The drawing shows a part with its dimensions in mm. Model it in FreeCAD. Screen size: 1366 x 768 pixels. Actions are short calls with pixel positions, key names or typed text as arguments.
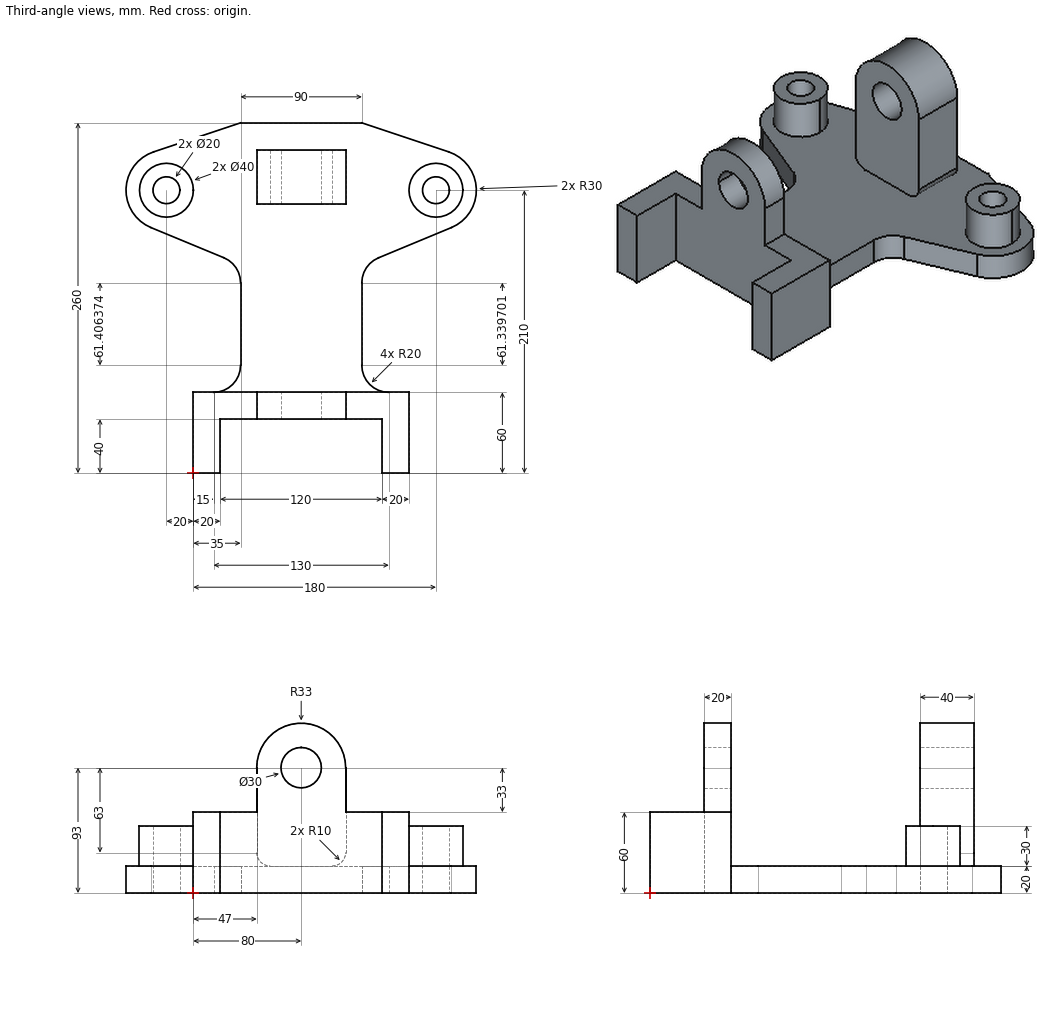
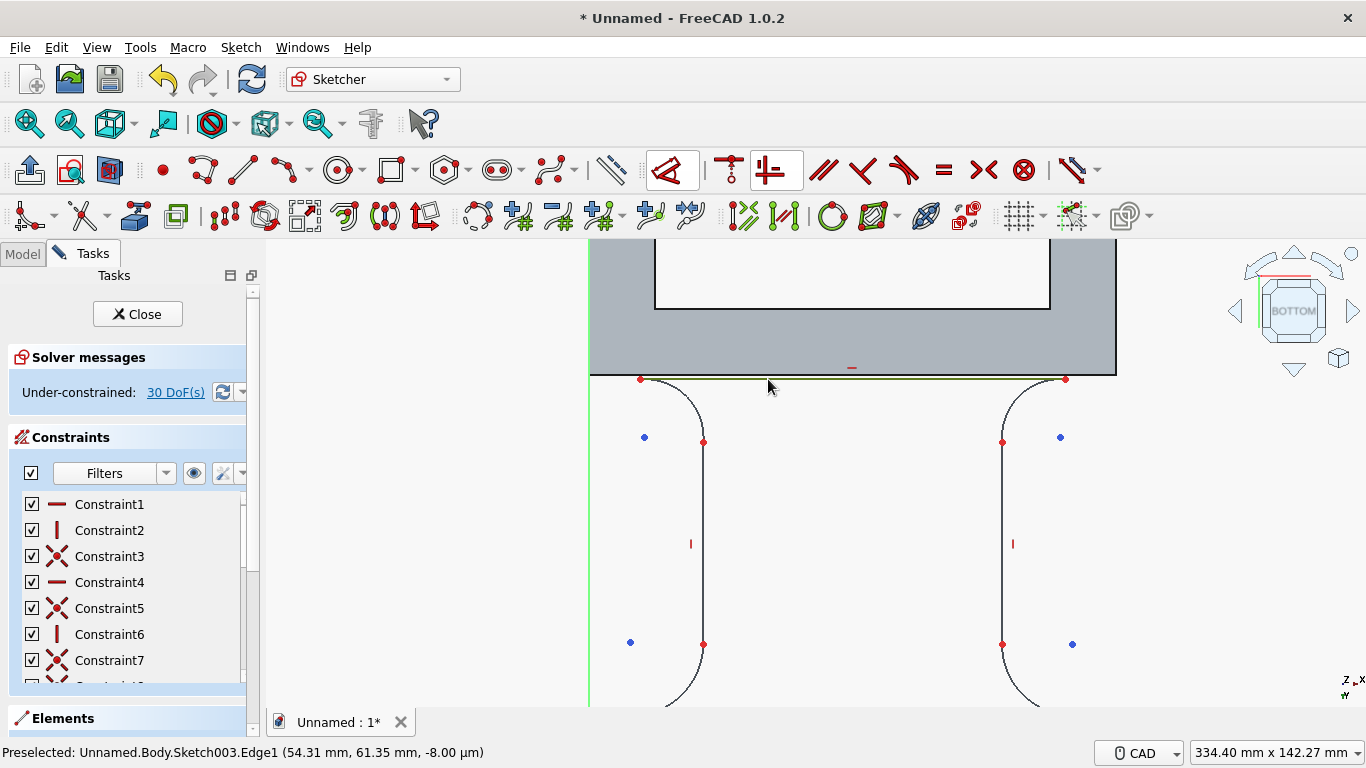
click(1007, 413)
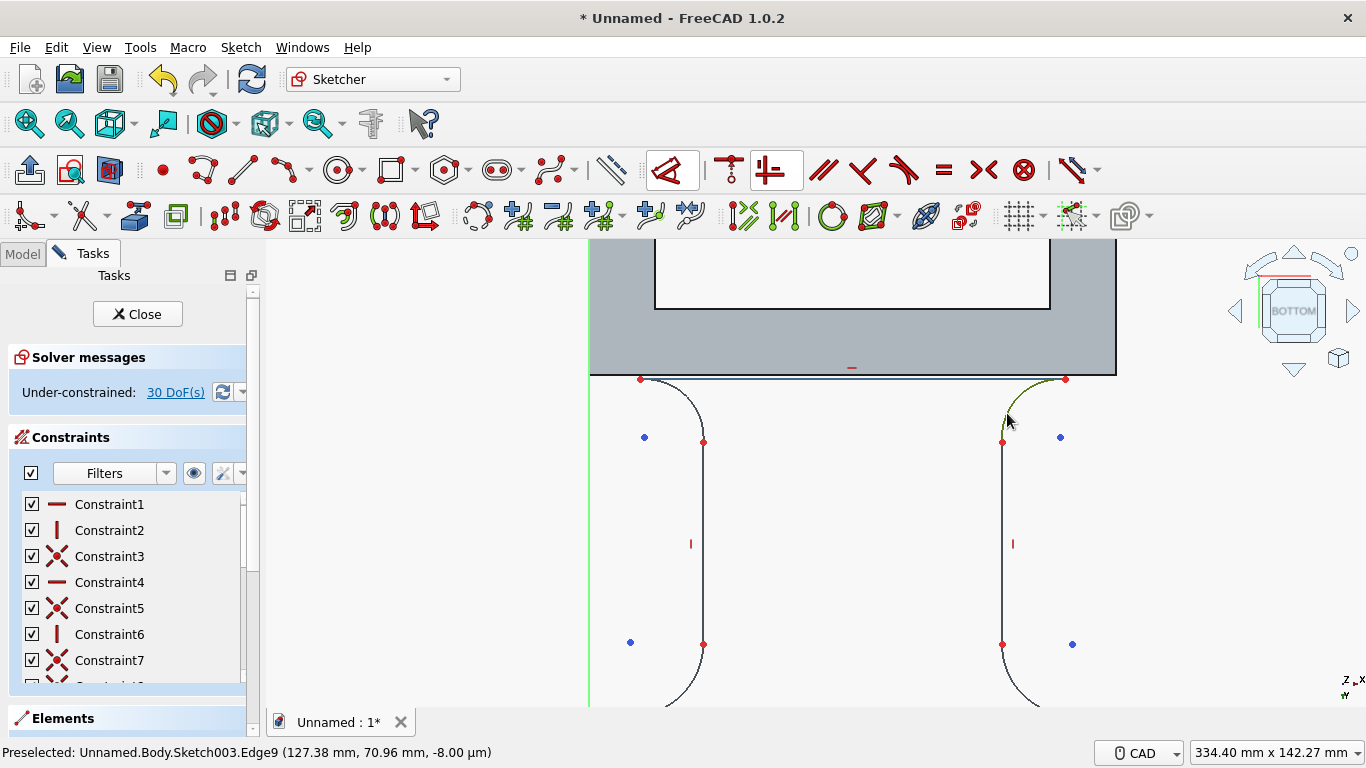
click(904, 170)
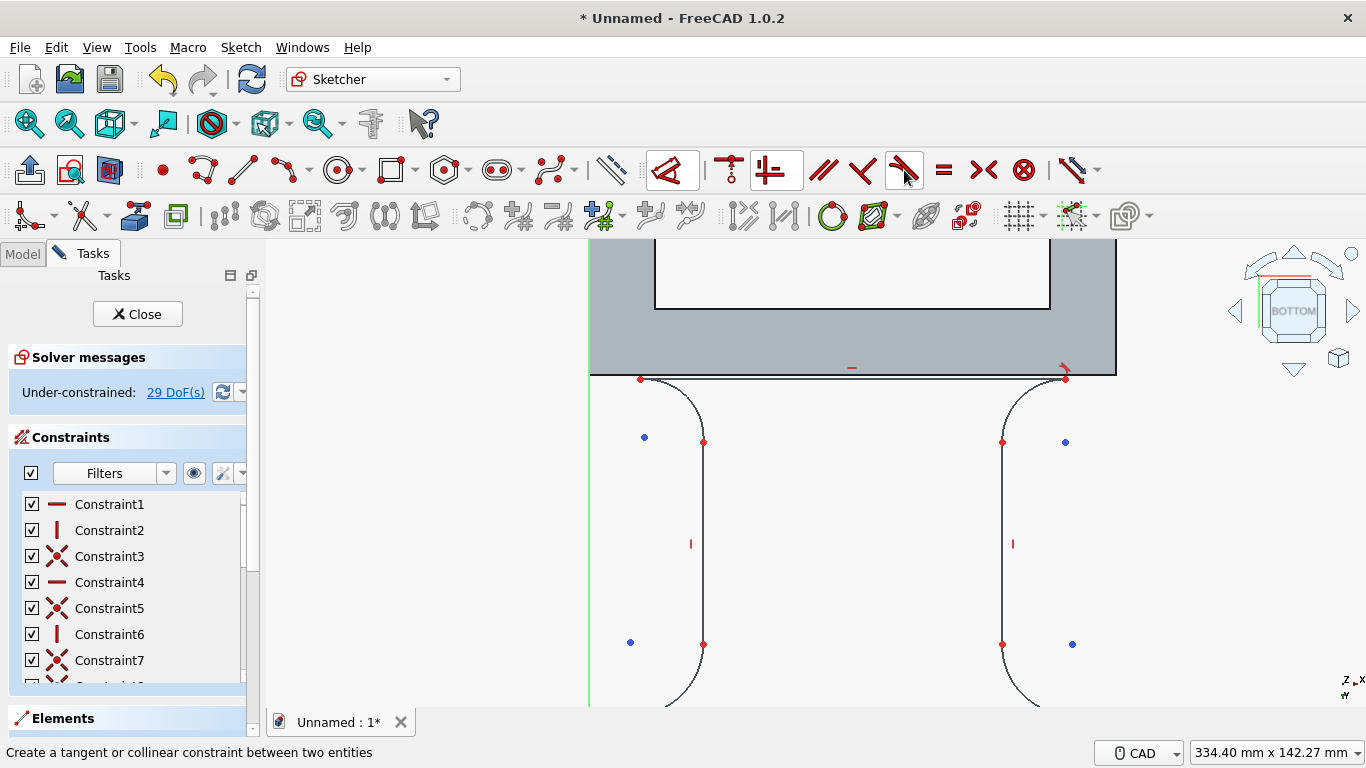
click(768, 379)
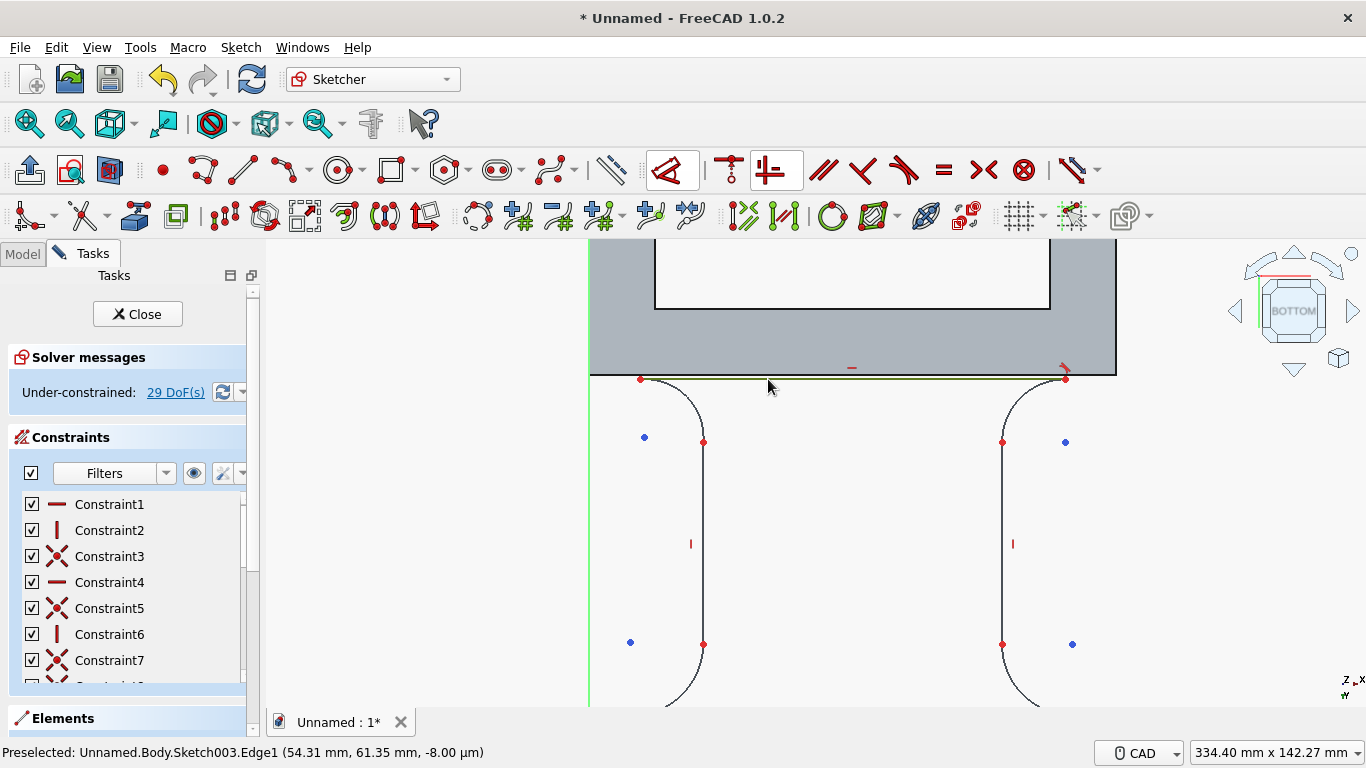
click(698, 413)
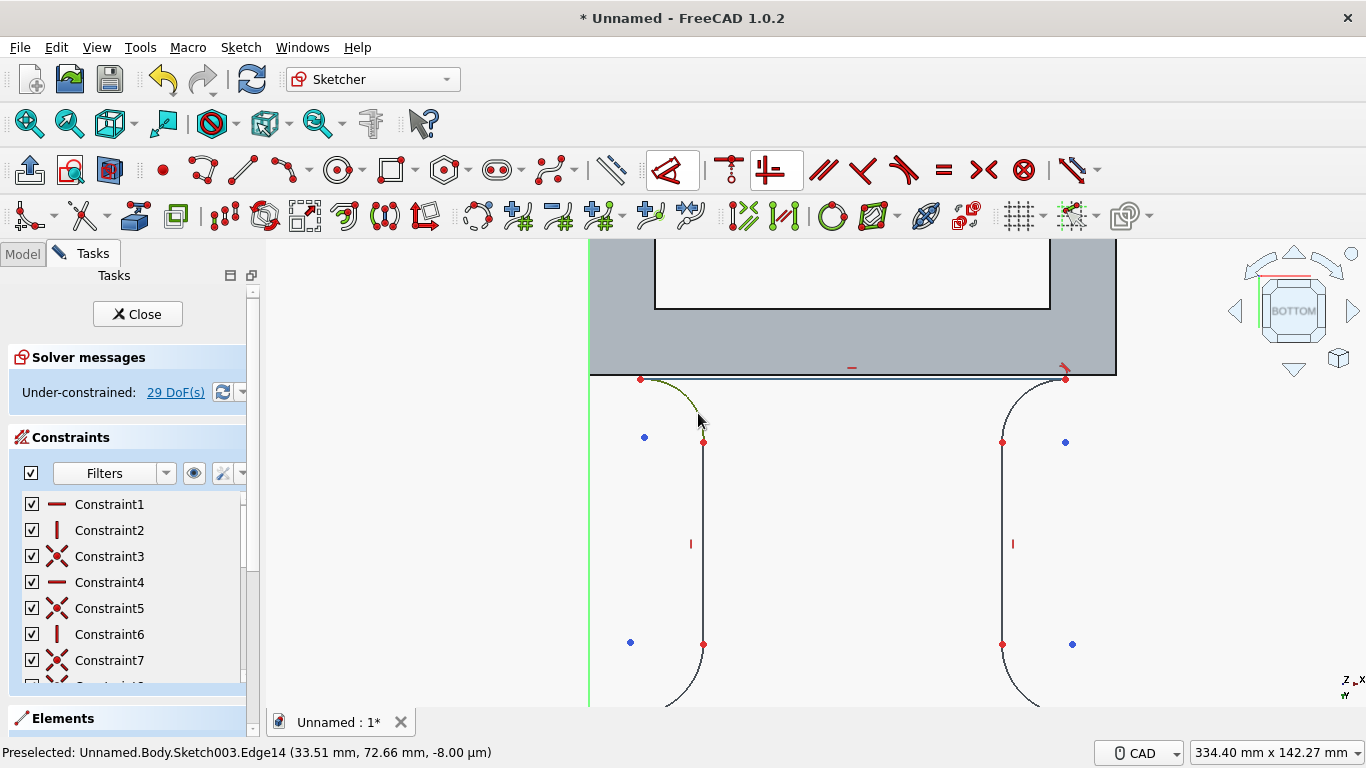
key(t)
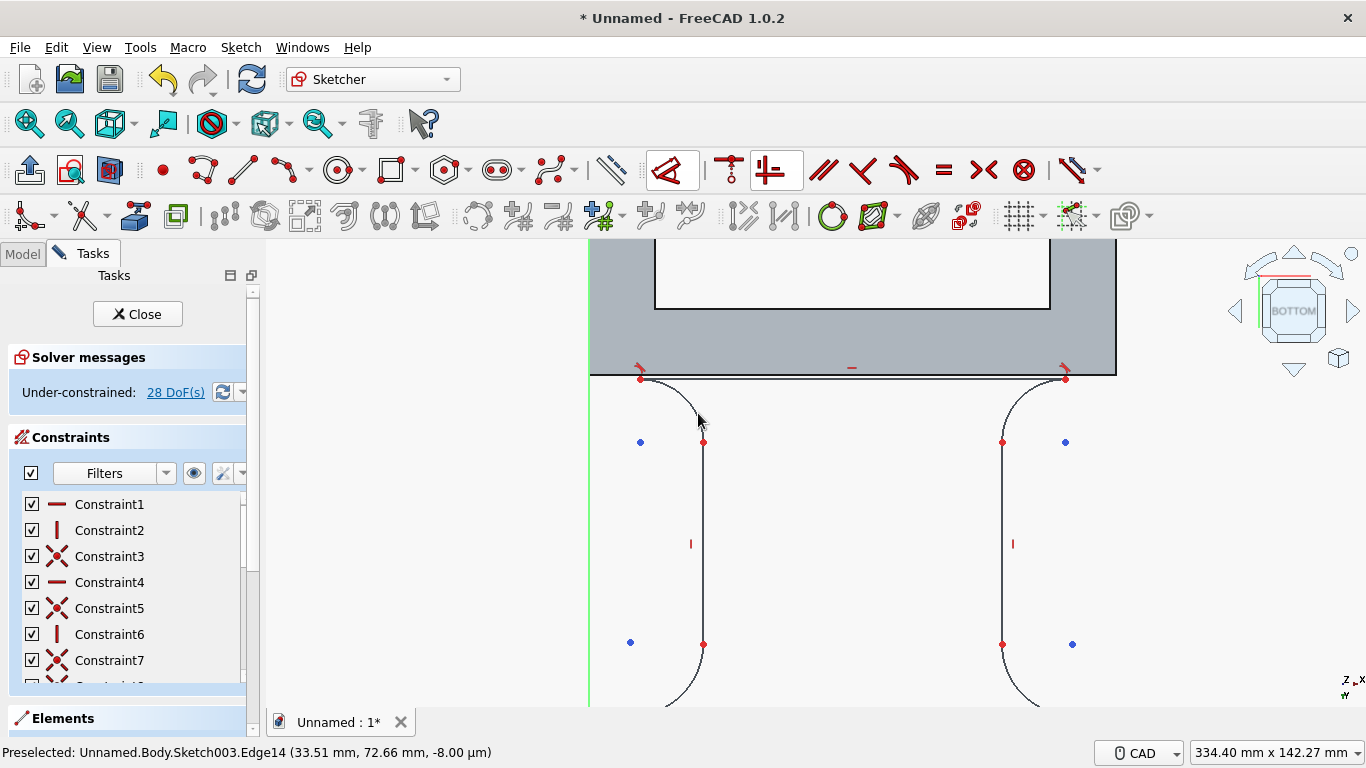
click(1002, 503)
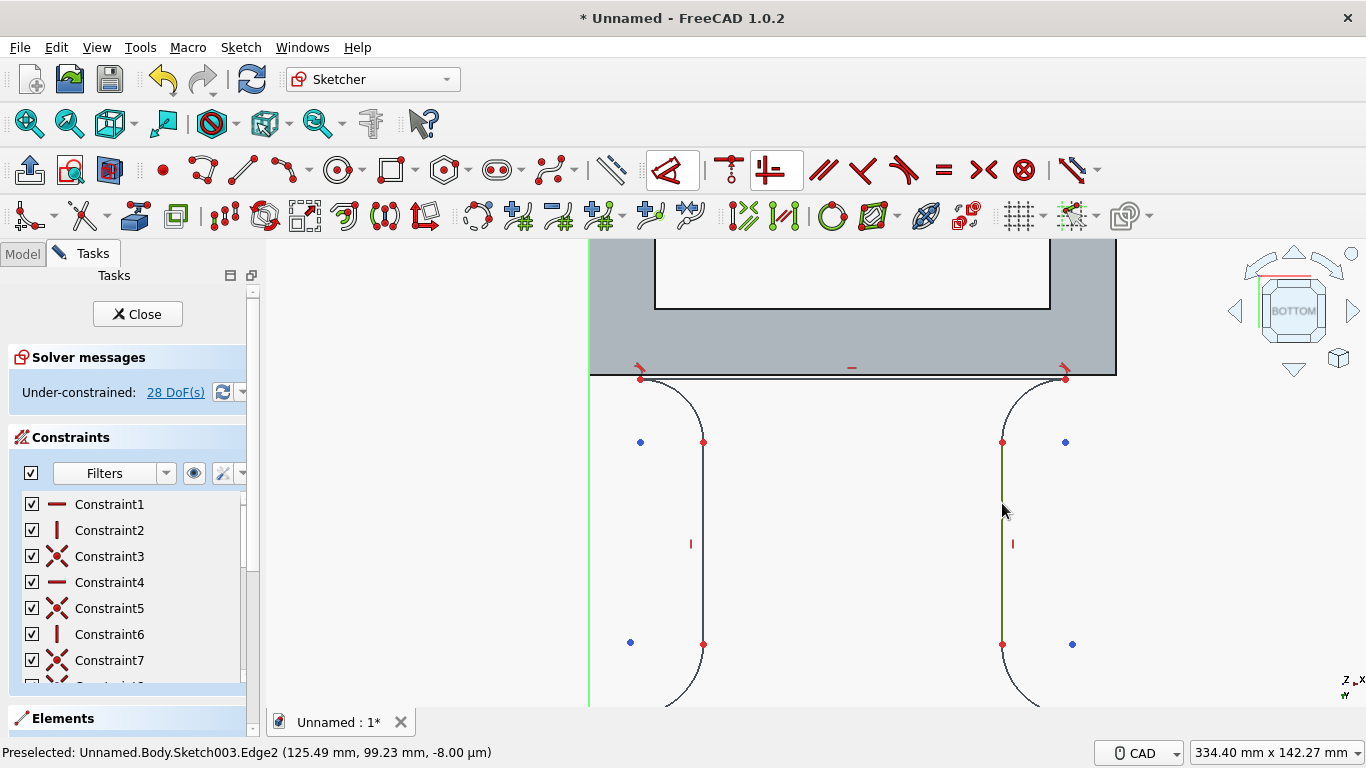
click(1009, 414)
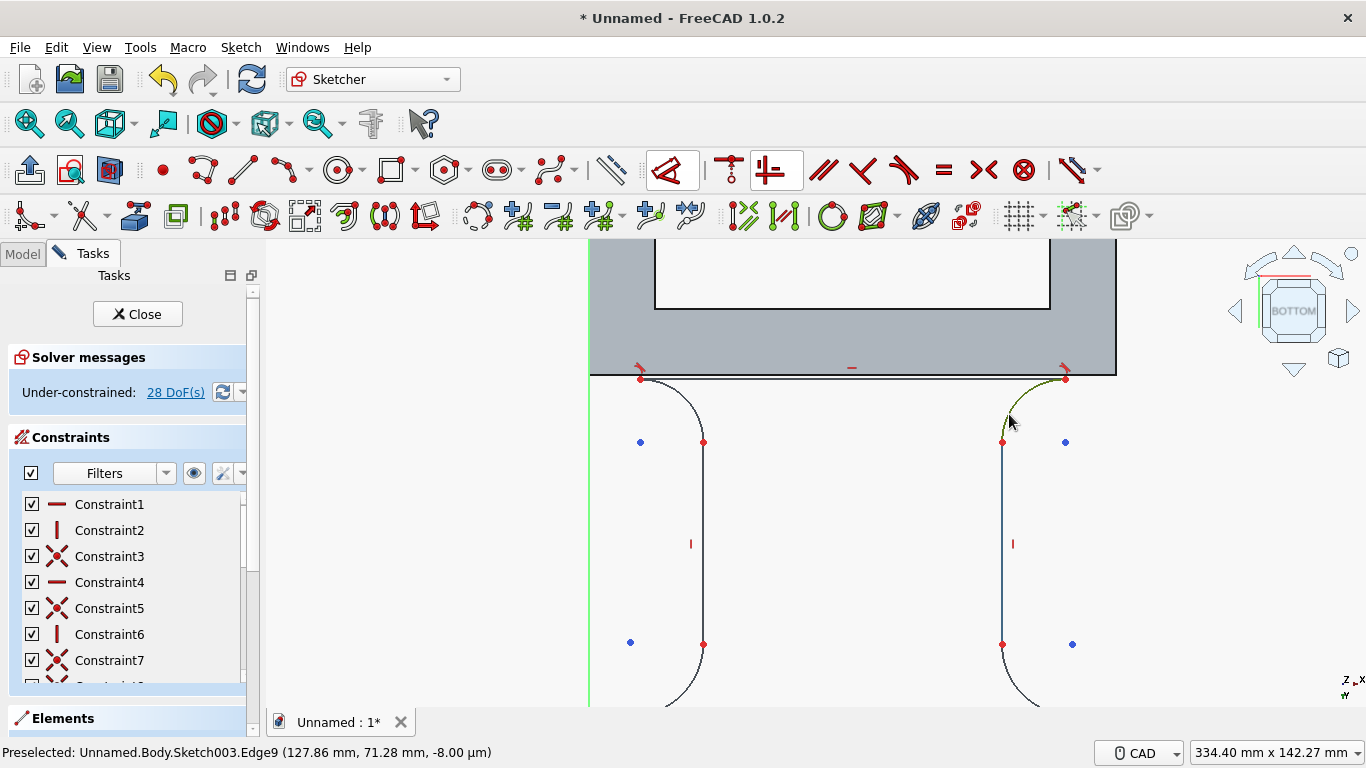
click(904, 170)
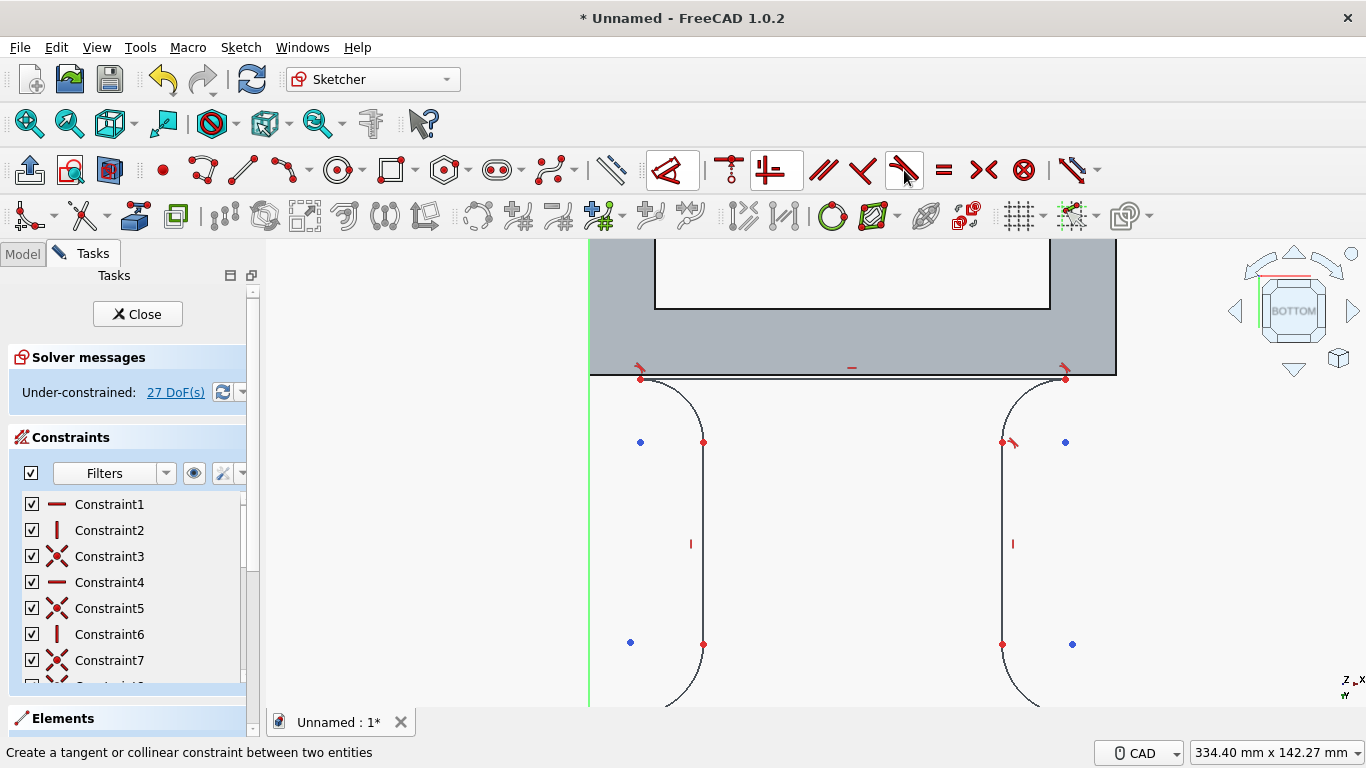
click(1002, 503)